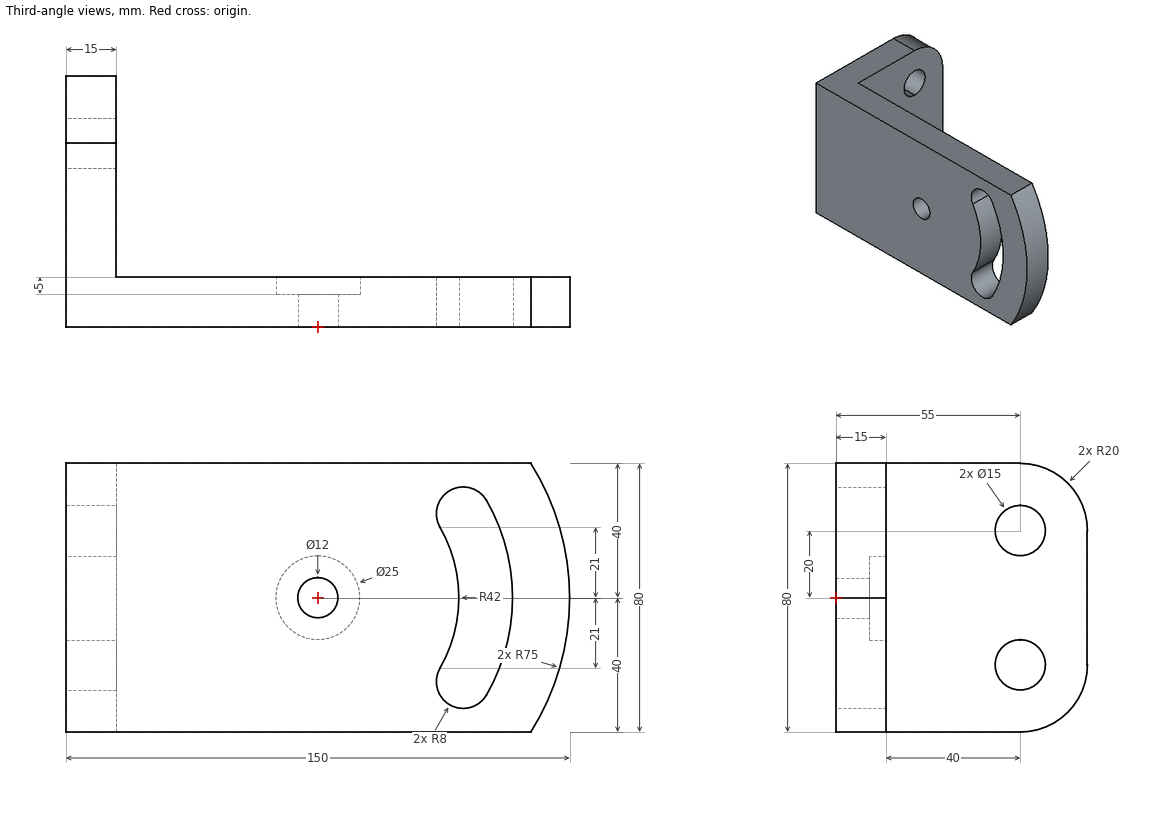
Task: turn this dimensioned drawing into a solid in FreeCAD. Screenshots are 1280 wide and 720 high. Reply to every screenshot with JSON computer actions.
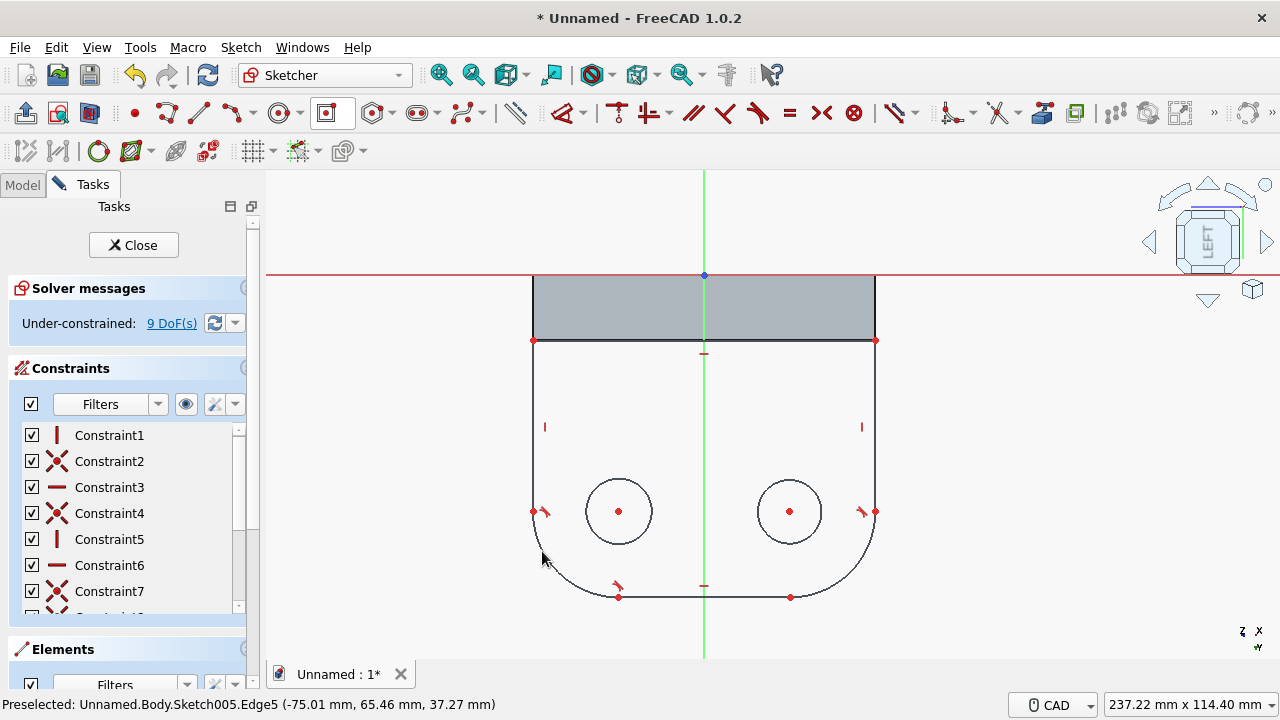
{"action": "left_click", "coordinate": [670, 597]}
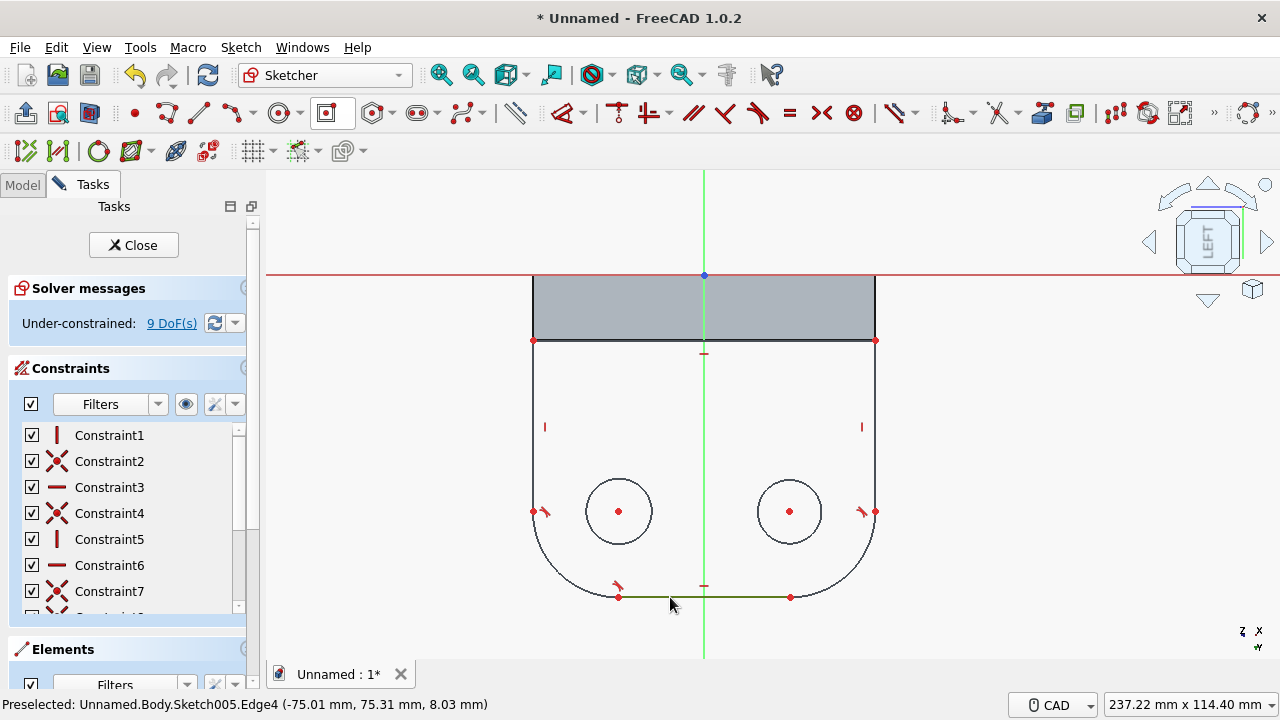
{"action": "left_click", "coordinate": [829, 588]}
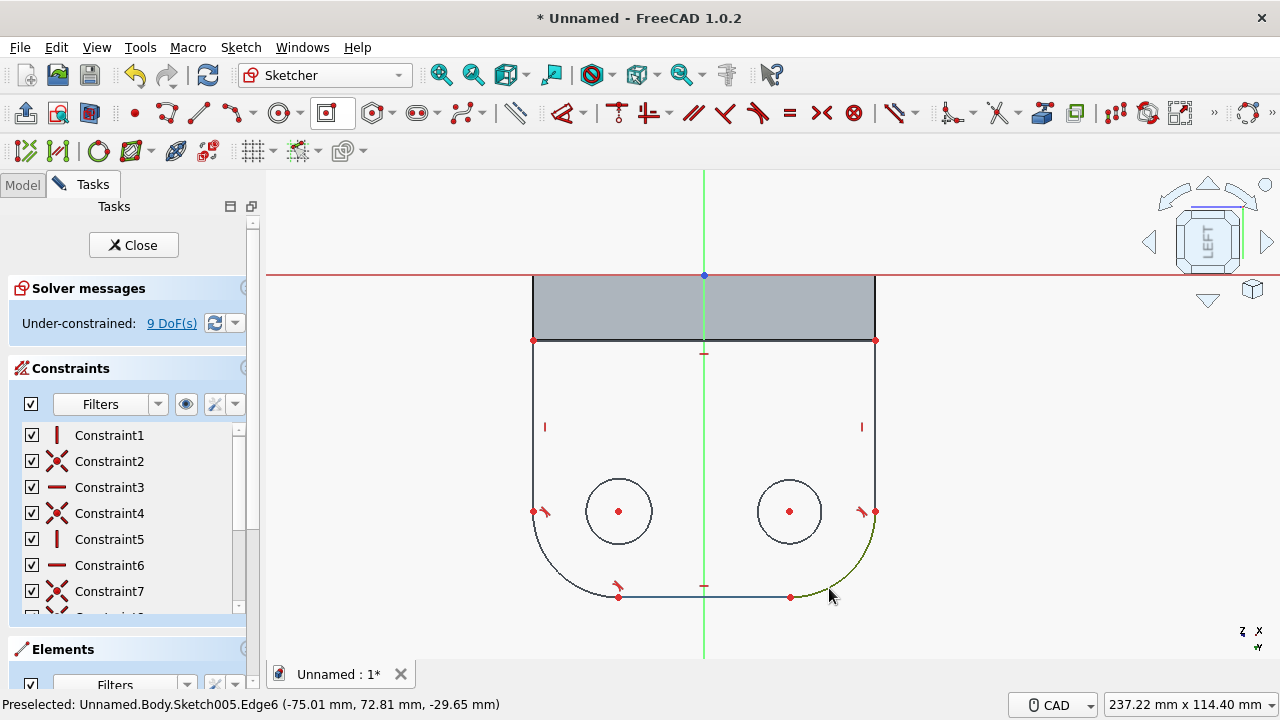
{"action": "left_click", "coordinate": [758, 114]}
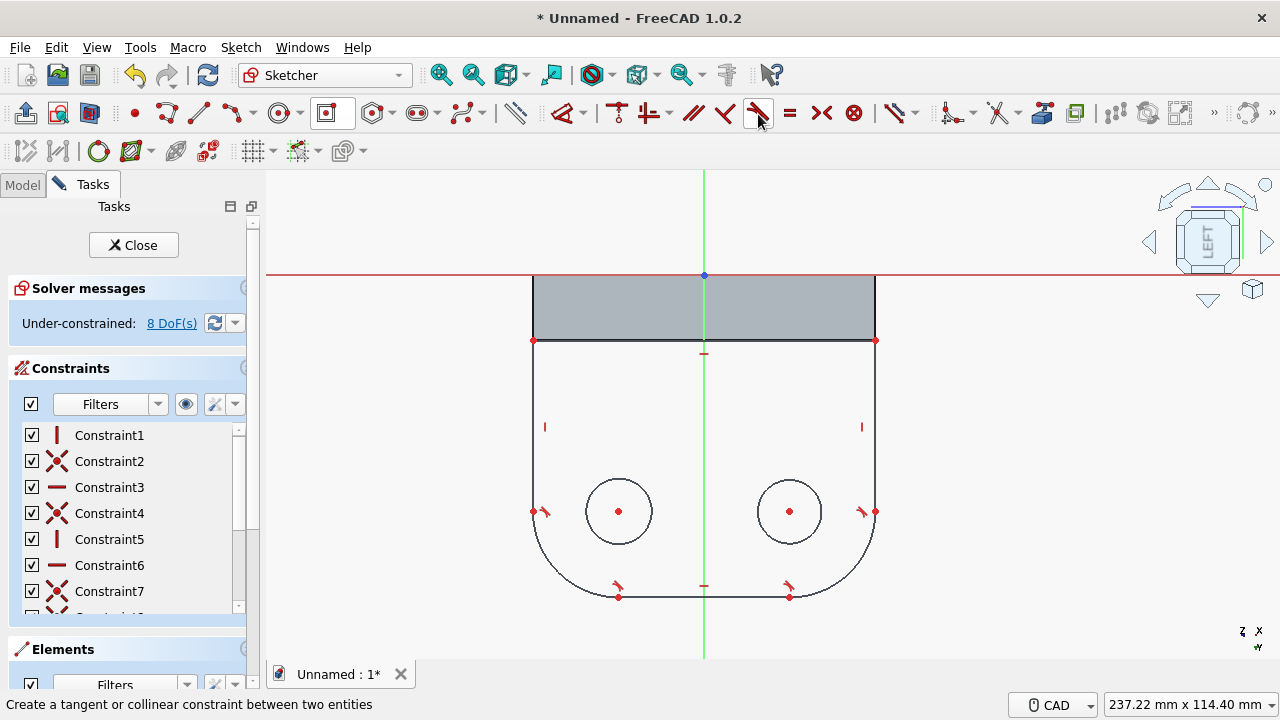
{"action": "left_click", "coordinate": [542, 550]}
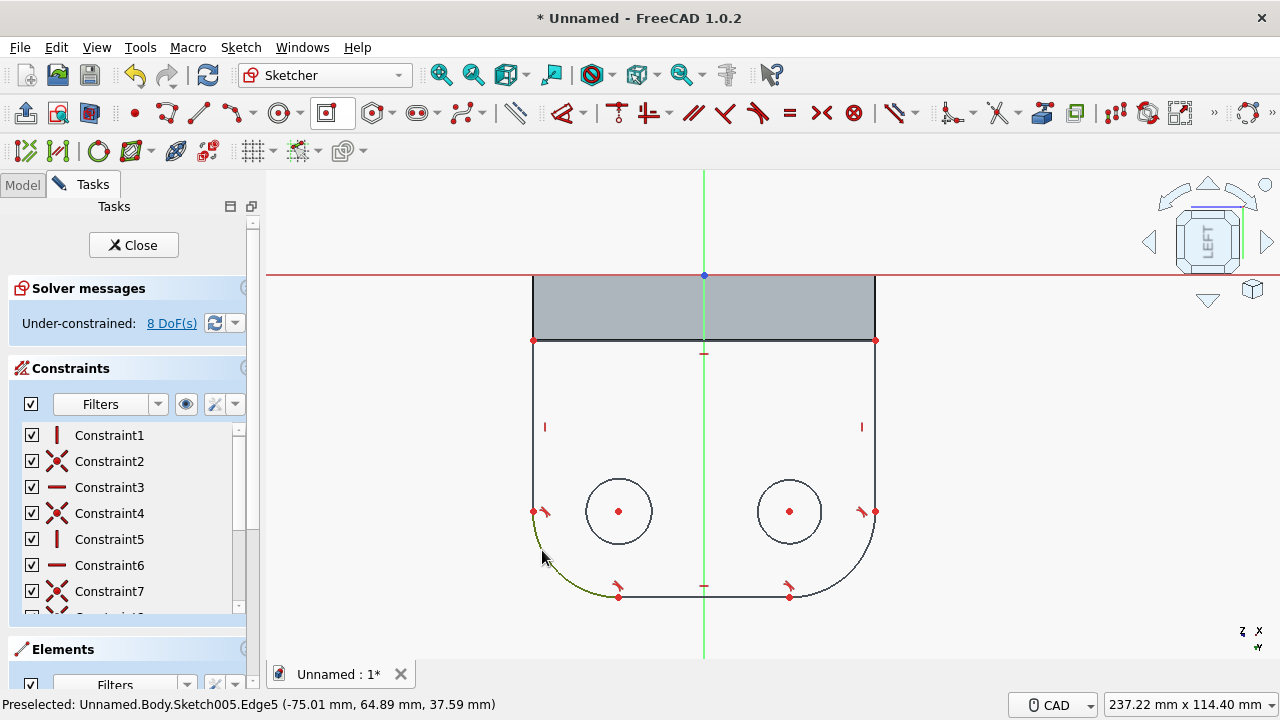
{"action": "left_click", "coordinate": [828, 588]}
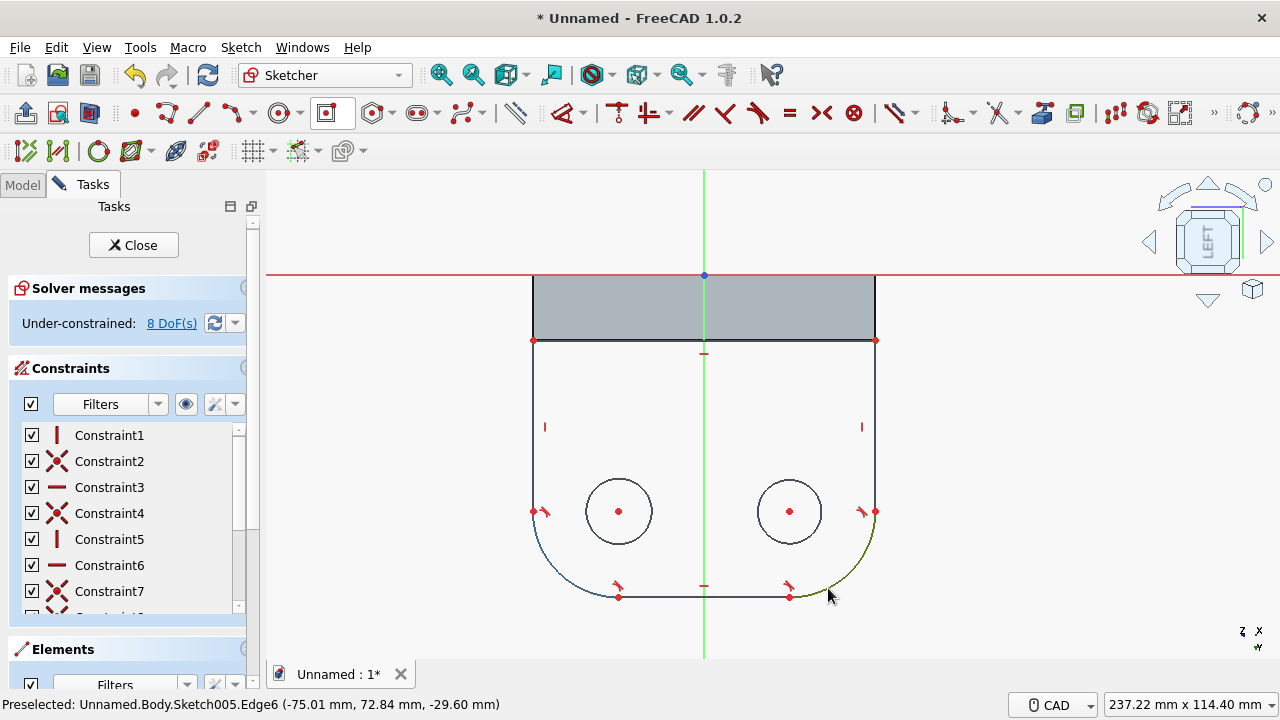
{"action": "left_click", "coordinate": [790, 114]}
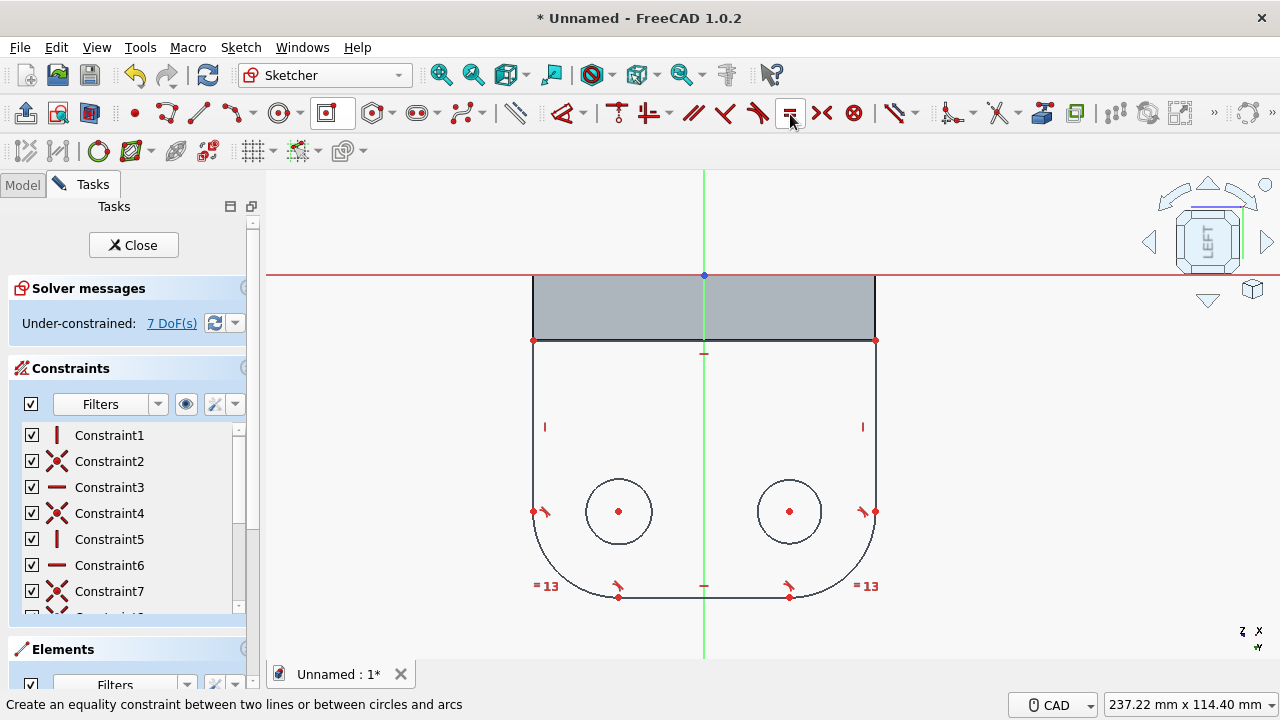
{"action": "left_click", "coordinate": [642, 489]}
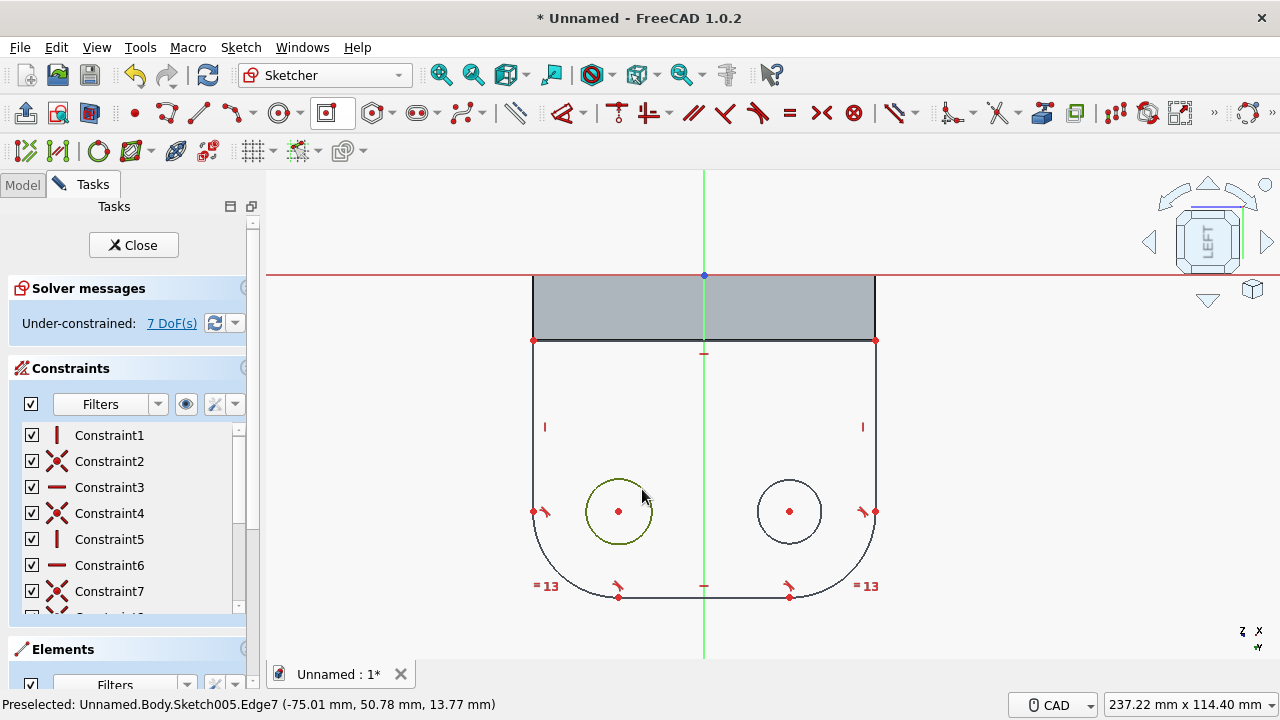
{"action": "left_click", "coordinate": [812, 489]}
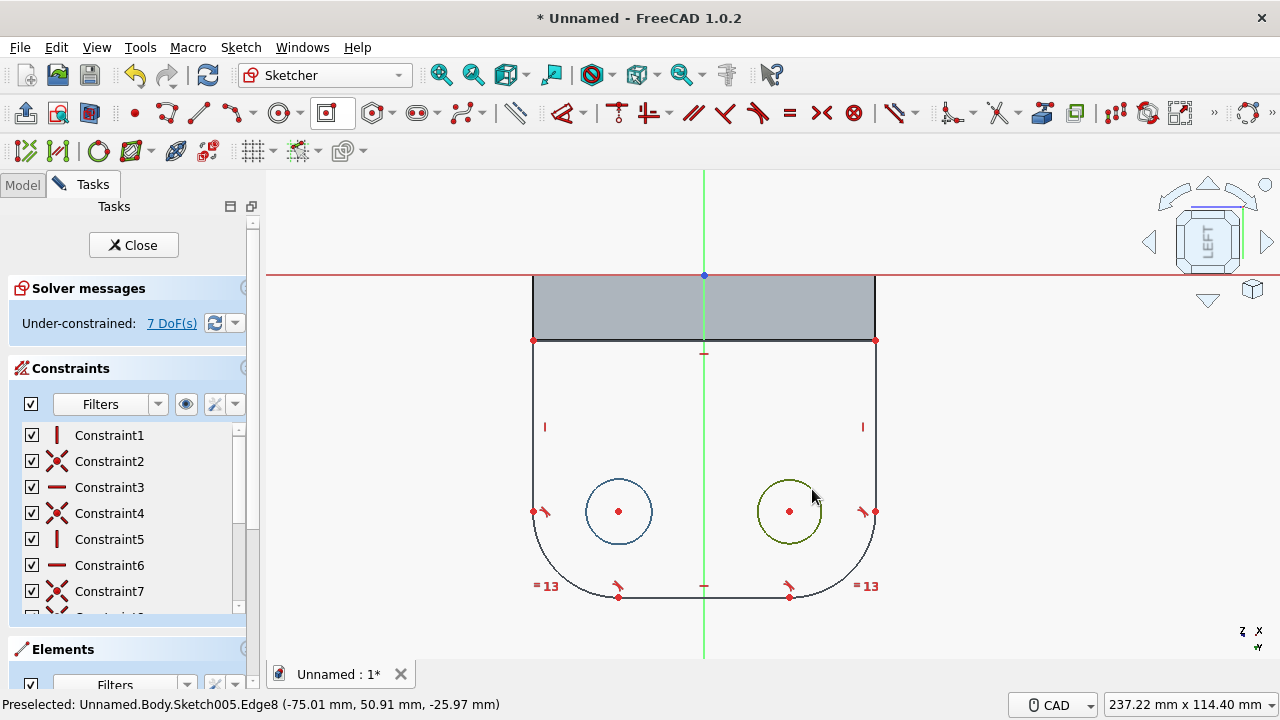
{"action": "key", "text": "e"}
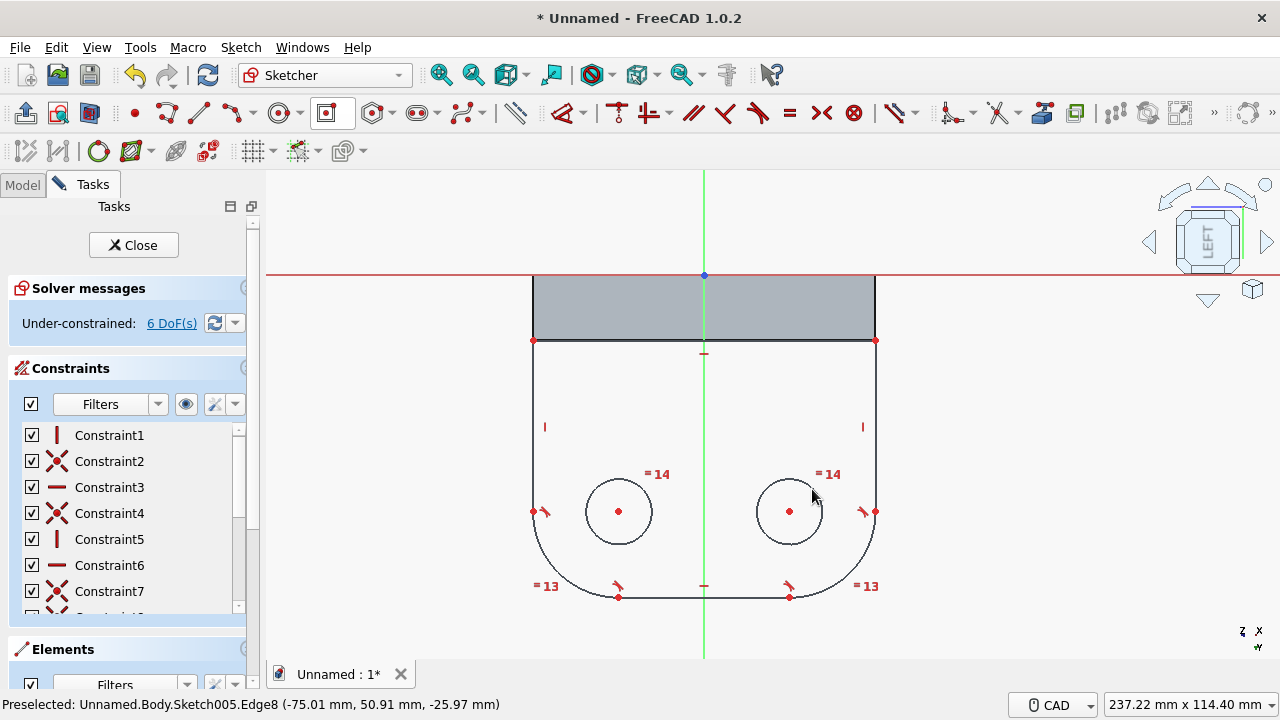
{"action": "left_click", "coordinate": [562, 114]}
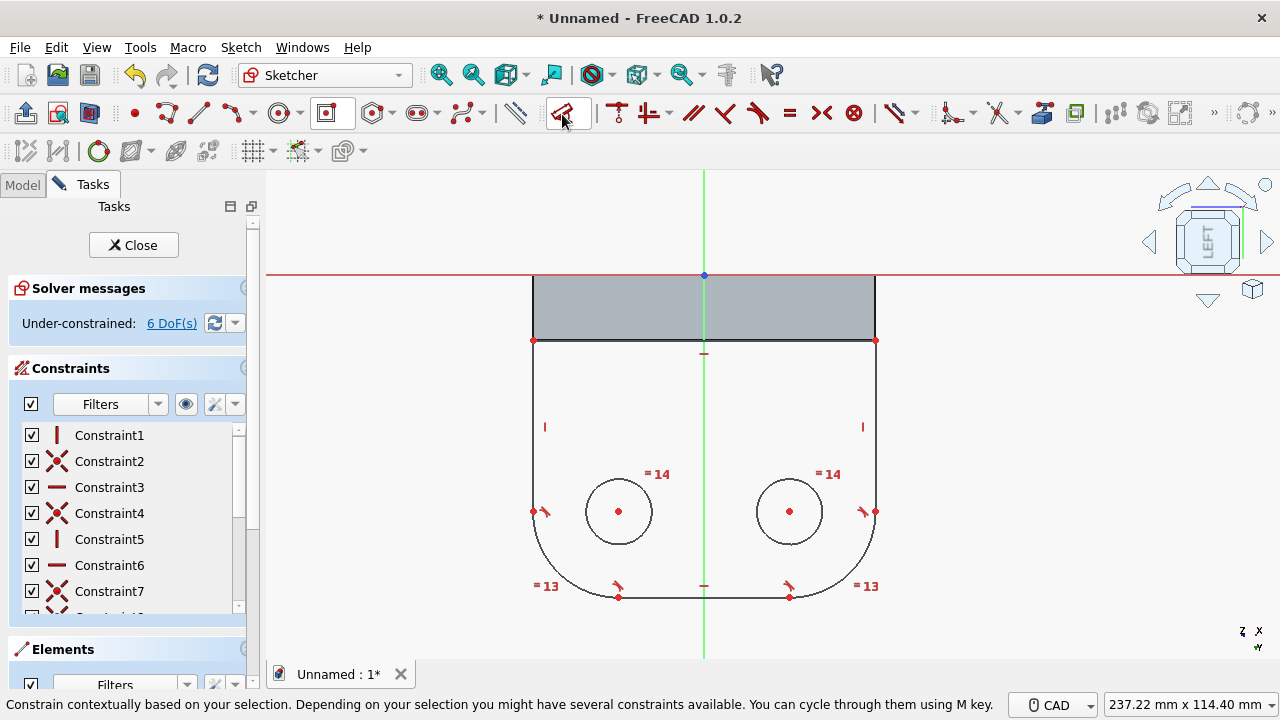
{"action": "left_click", "coordinate": [542, 551]}
{"action": "left_click", "coordinate": [513, 566]}